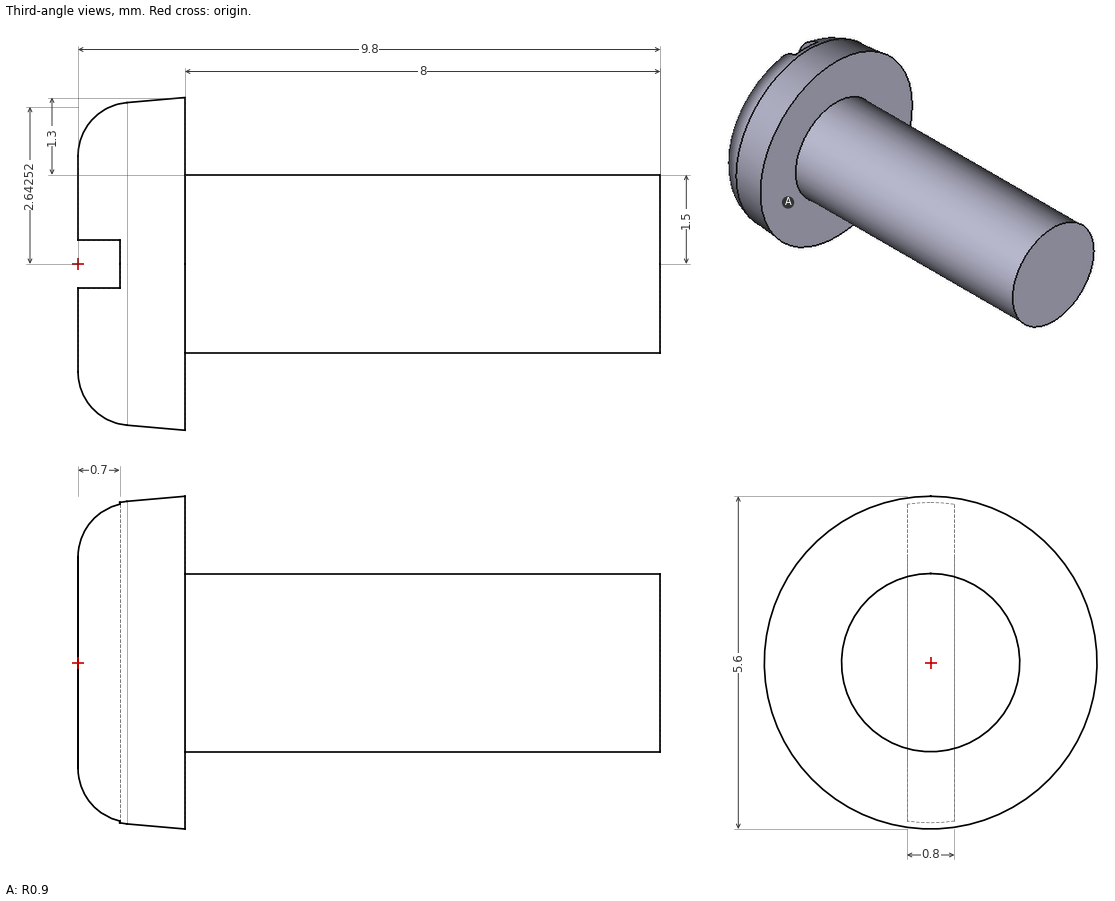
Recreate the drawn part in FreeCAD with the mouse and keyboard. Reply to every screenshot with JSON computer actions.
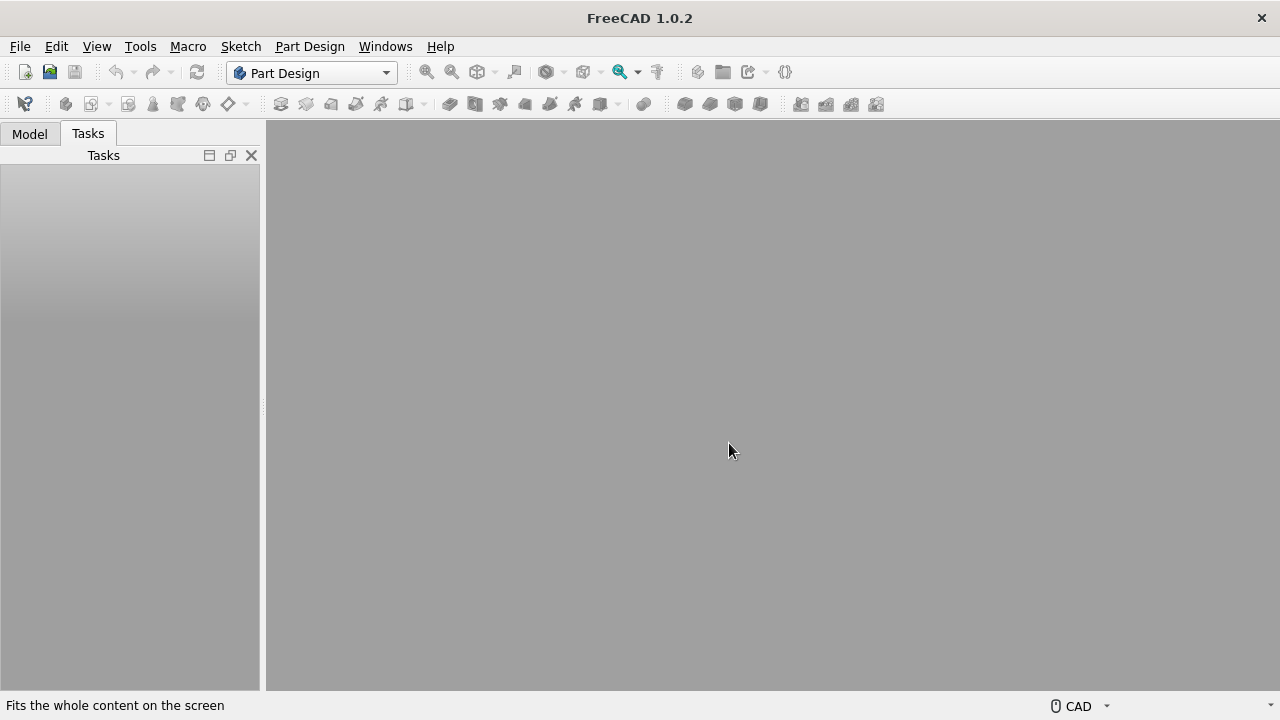
{"action": "left_click", "coordinate": [25, 72]}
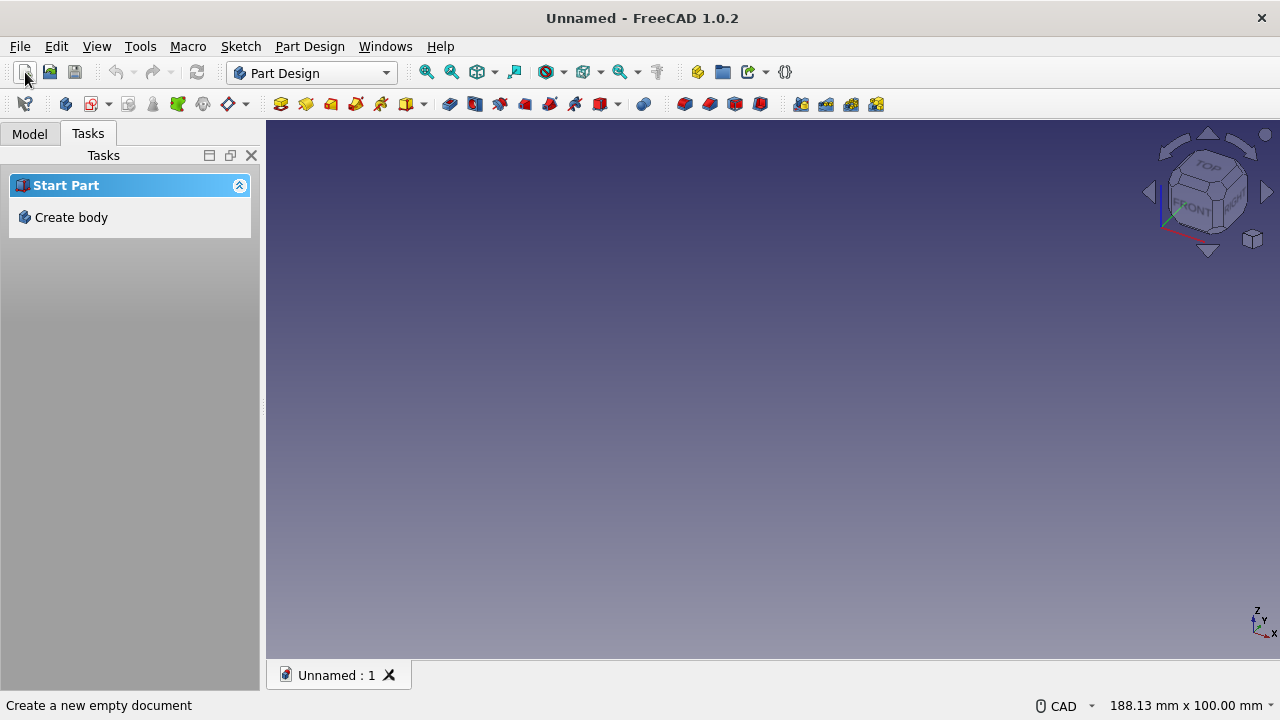
{"action": "left_click", "coordinate": [90, 104]}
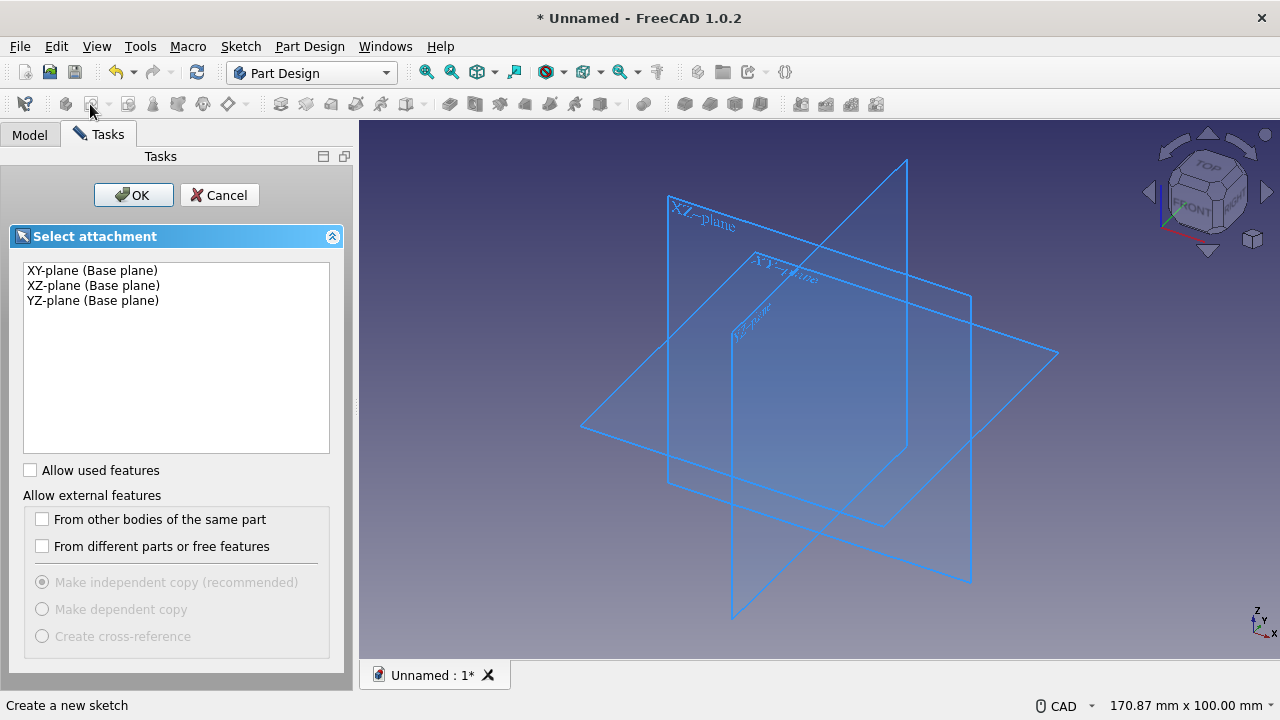
{"action": "left_click", "coordinate": [84, 270]}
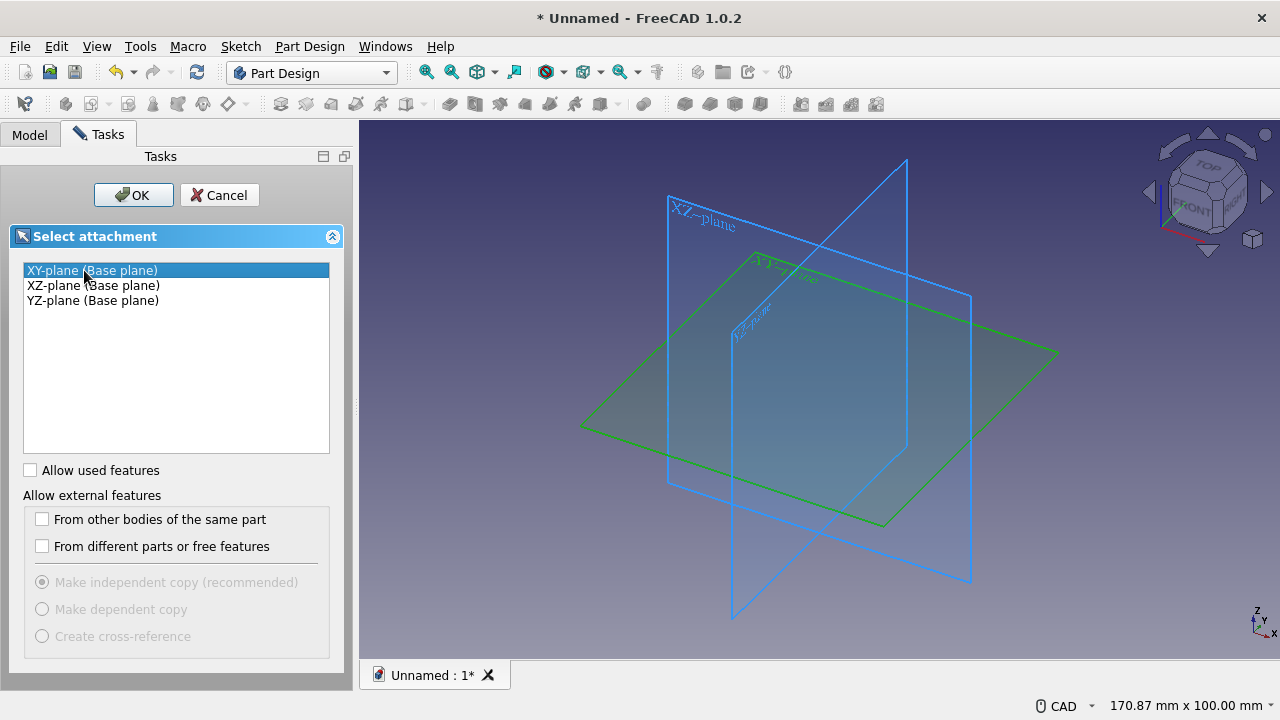
{"action": "left_click", "coordinate": [134, 195]}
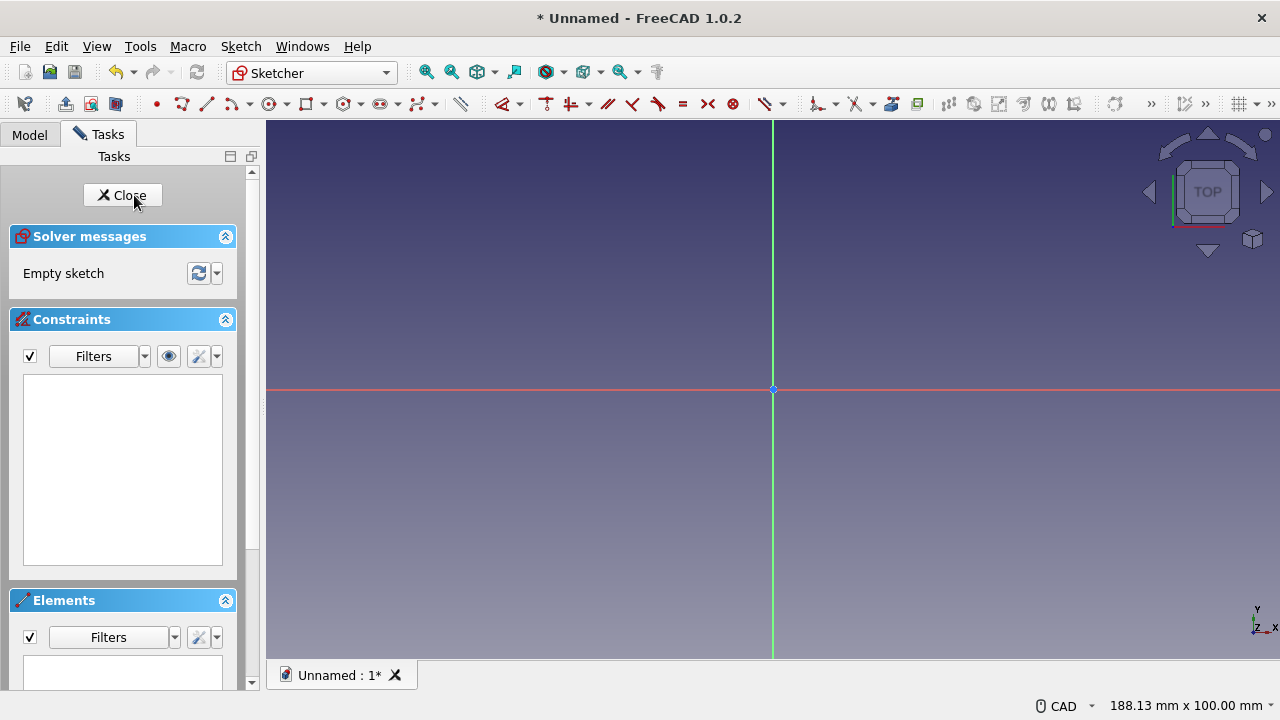
{"action": "scroll", "coordinate": [809, 381], "scroll_direction": "up", "scroll_amount": 12}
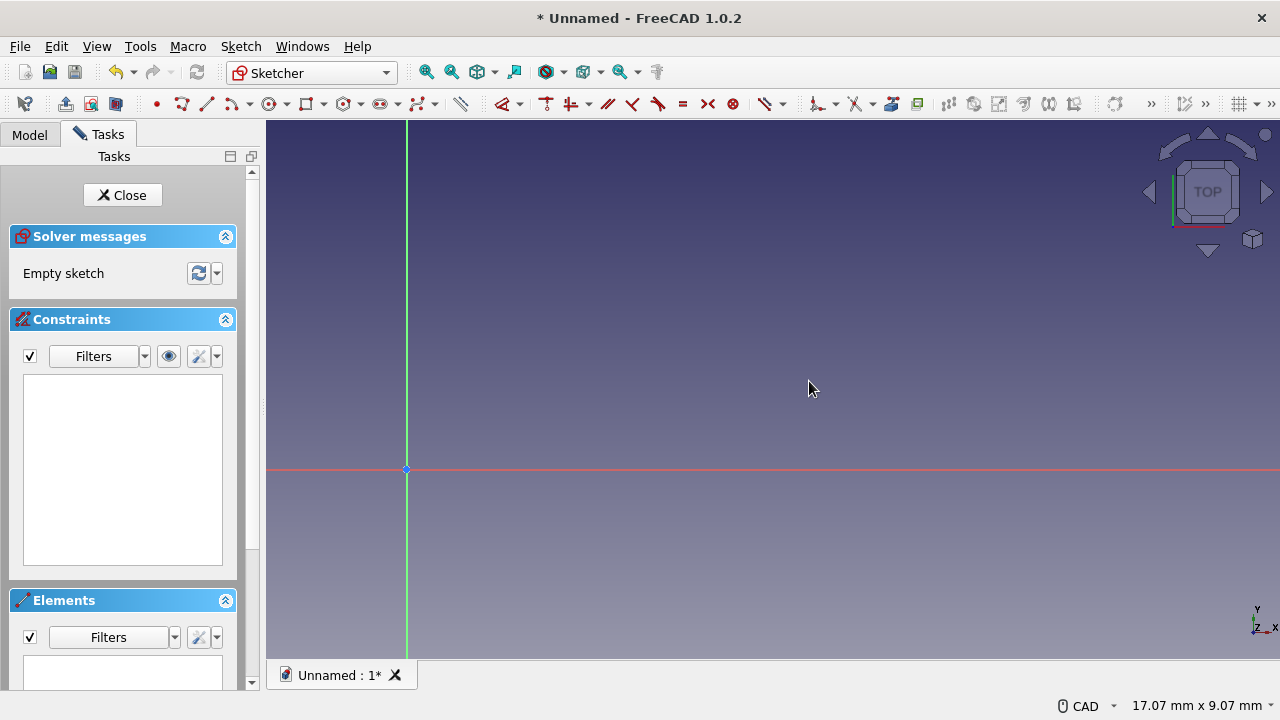
{"action": "left_click", "coordinate": [182, 104]}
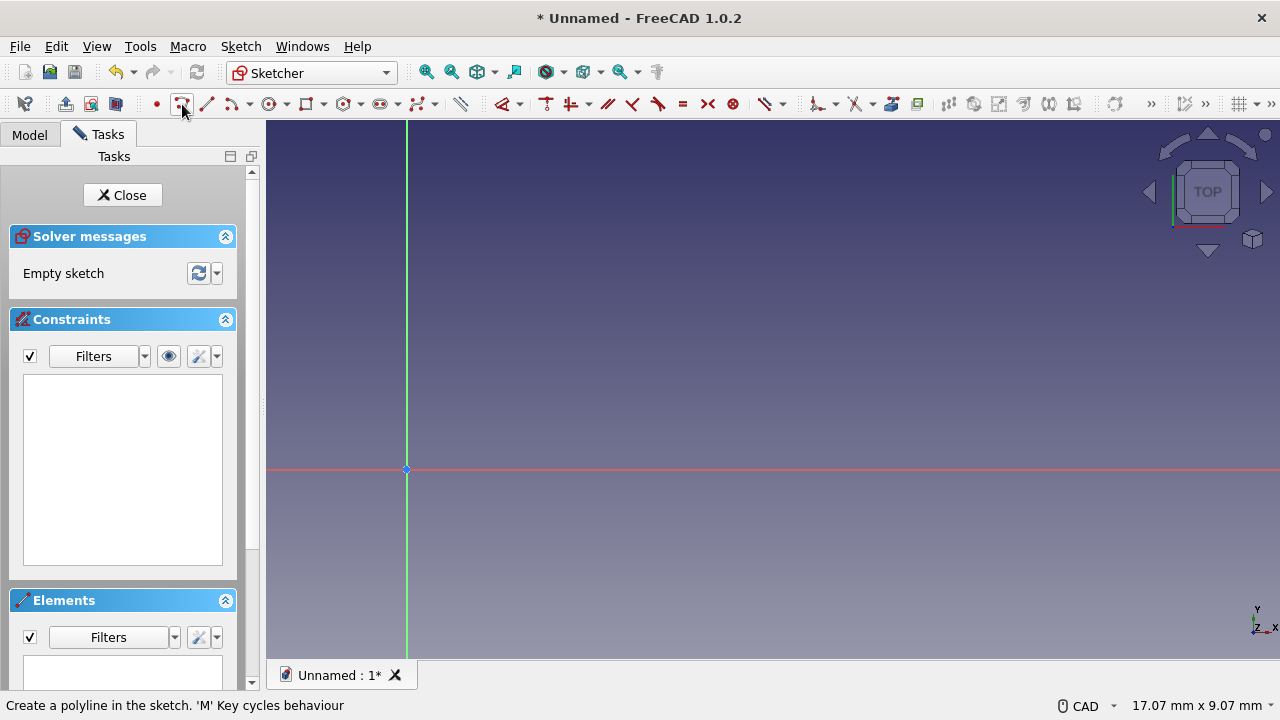
{"action": "left_click", "coordinate": [407, 470]}
{"action": "left_click", "coordinate": [989, 461]}
{"action": "left_click", "coordinate": [989, 381]}
{"action": "left_click", "coordinate": [514, 381]}
{"action": "left_click", "coordinate": [514, 303]}
{"action": "left_click", "coordinate": [416, 313]}
{"action": "left_click", "coordinate": [407, 470]}
{"action": "key", "text": "Escape"}
{"action": "key", "text": "Escape"}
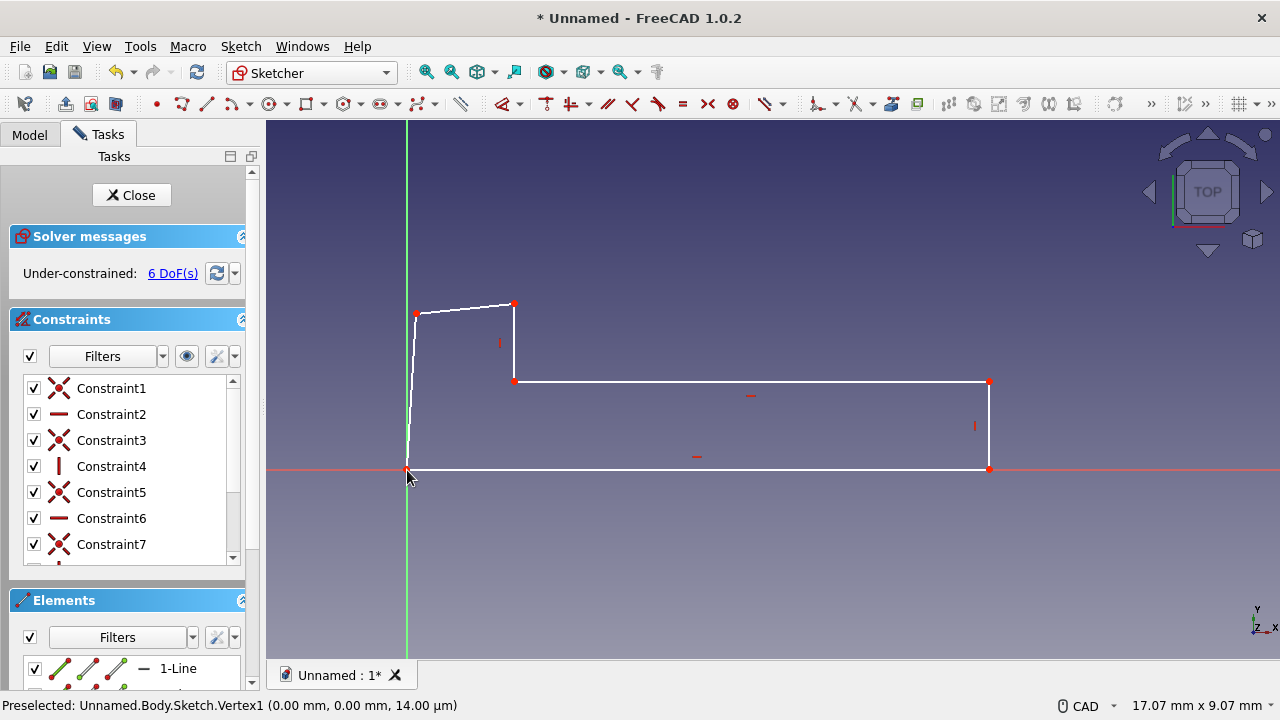
{"action": "left_click", "coordinate": [410, 423]}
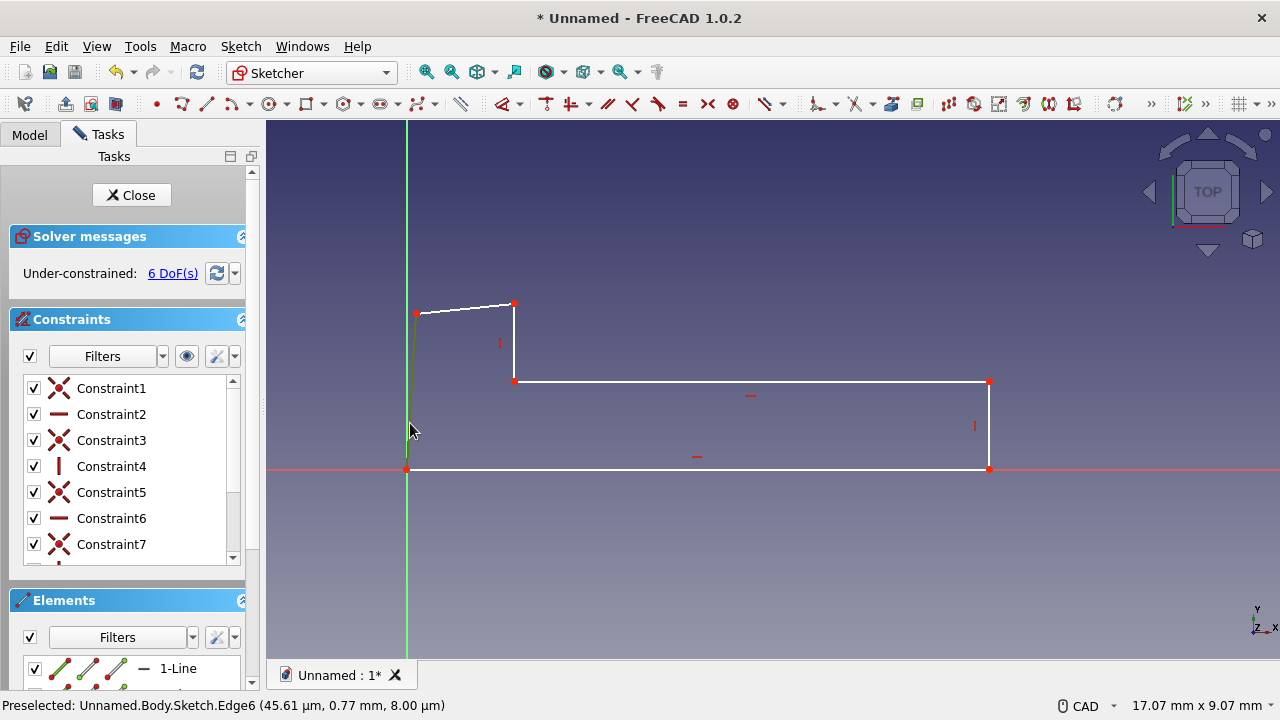
{"action": "left_click", "coordinate": [588, 104]}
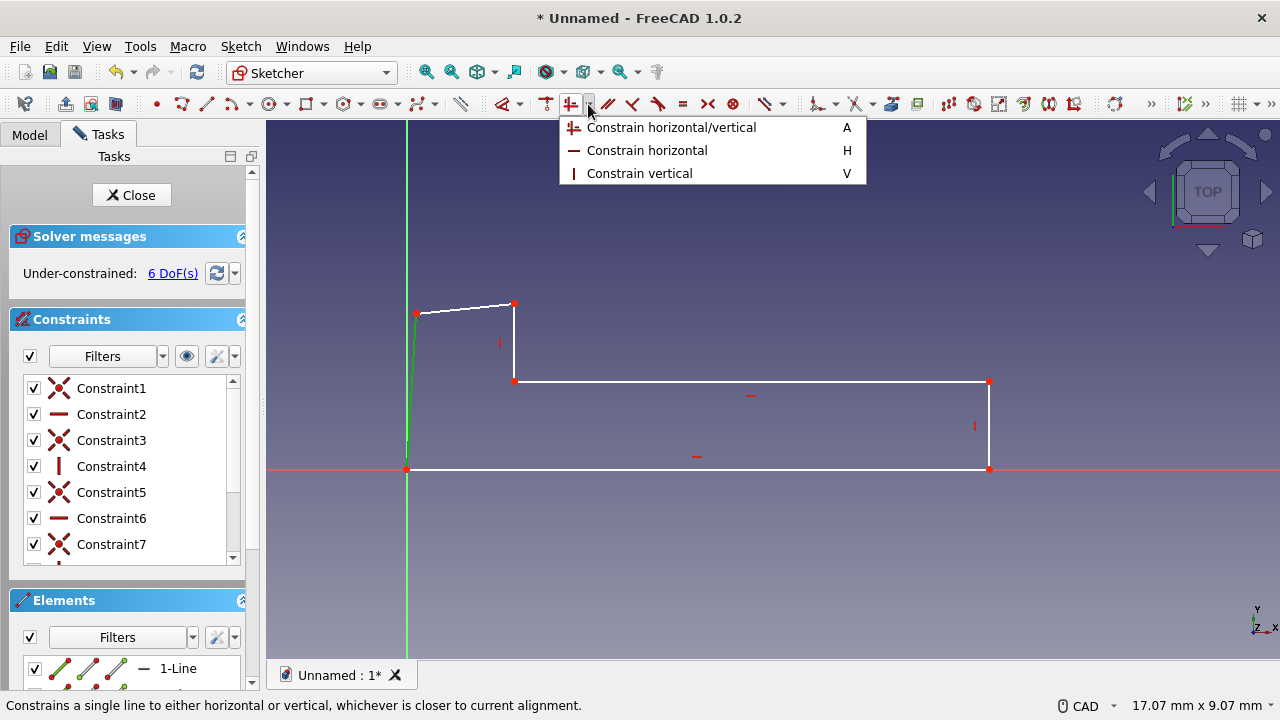
{"action": "left_click", "coordinate": [713, 174]}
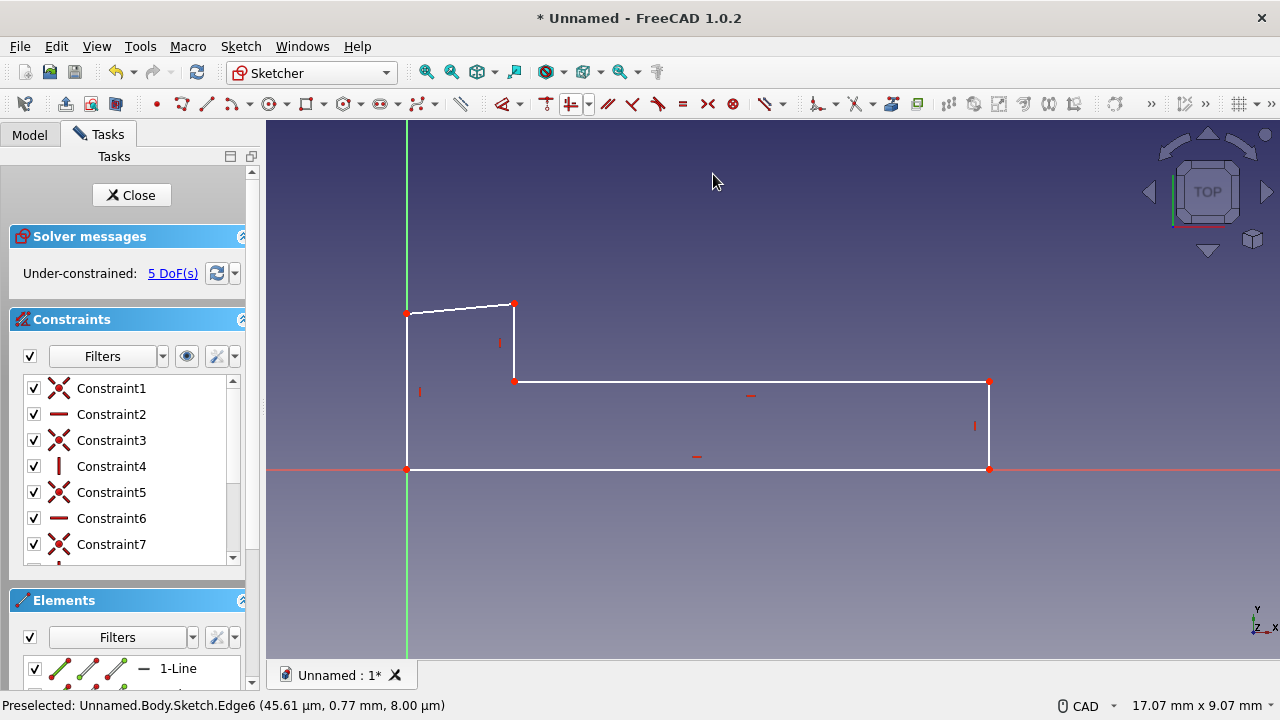
{"action": "left_click", "coordinate": [847, 382]}